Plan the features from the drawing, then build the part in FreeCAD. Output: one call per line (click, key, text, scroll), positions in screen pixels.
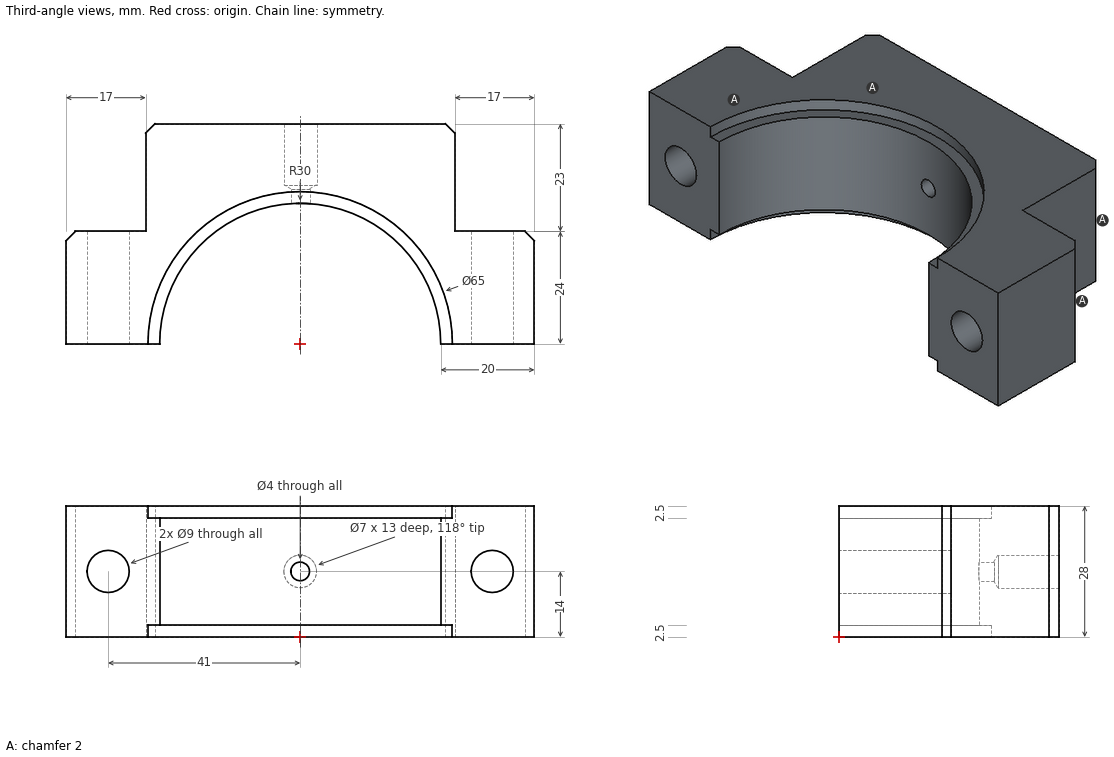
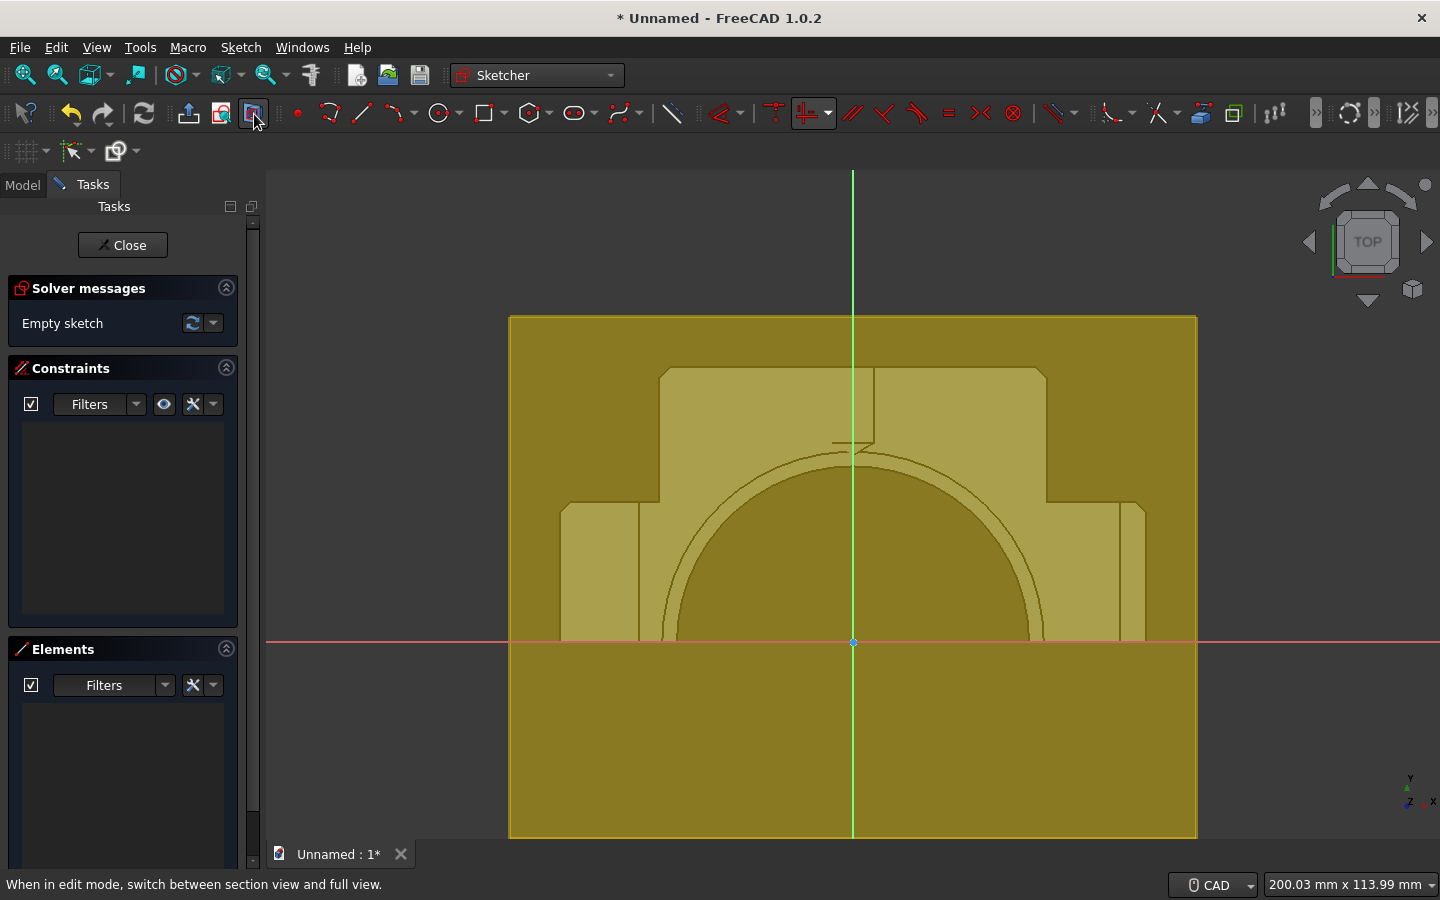
scroll(475, 198, down, 1)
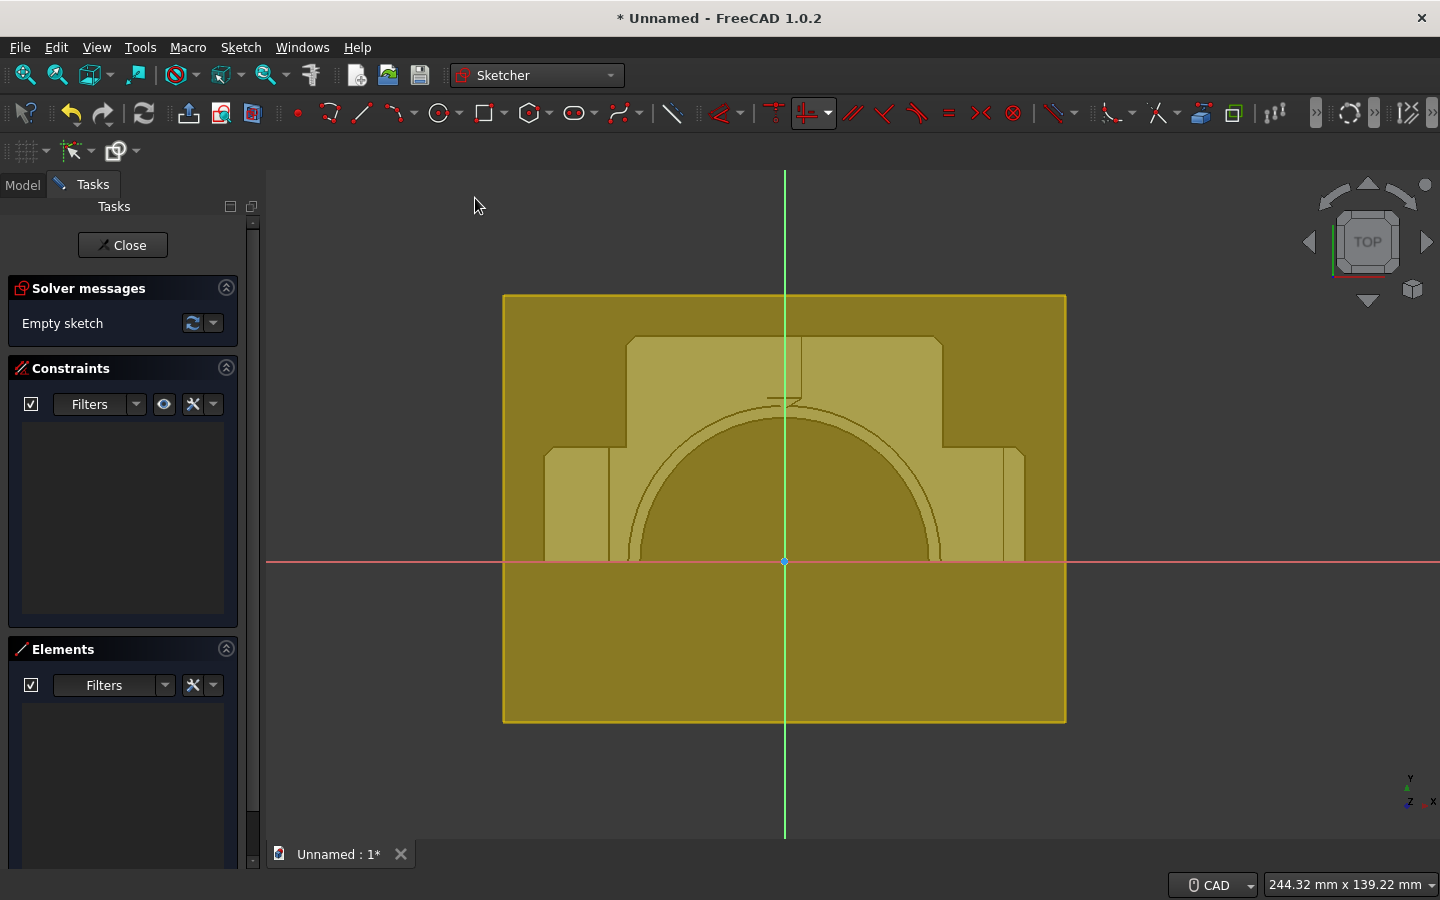
scroll(785, 679, up, 2)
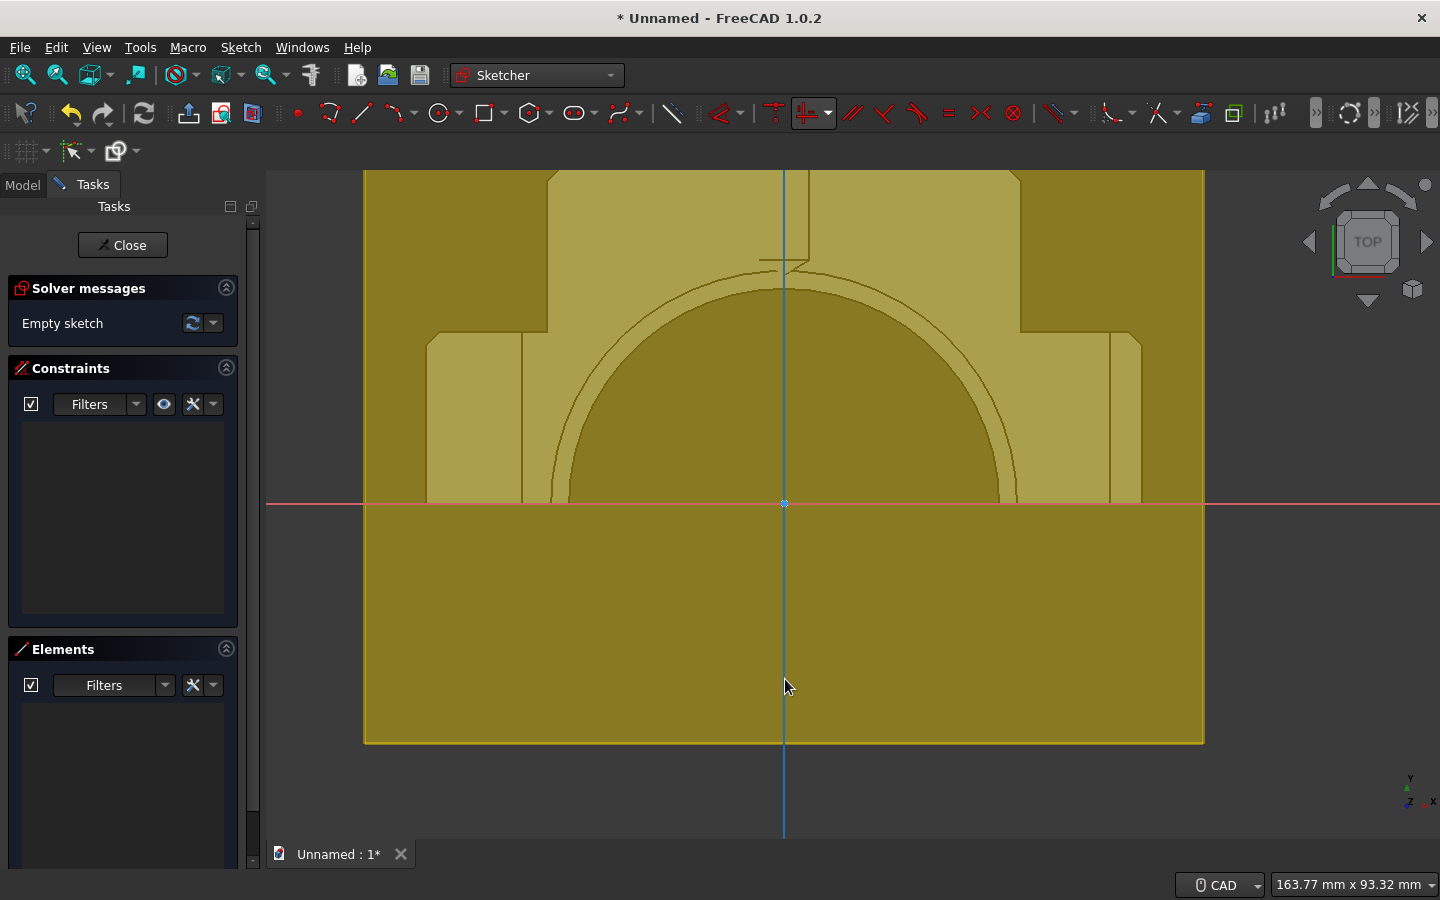
click(440, 114)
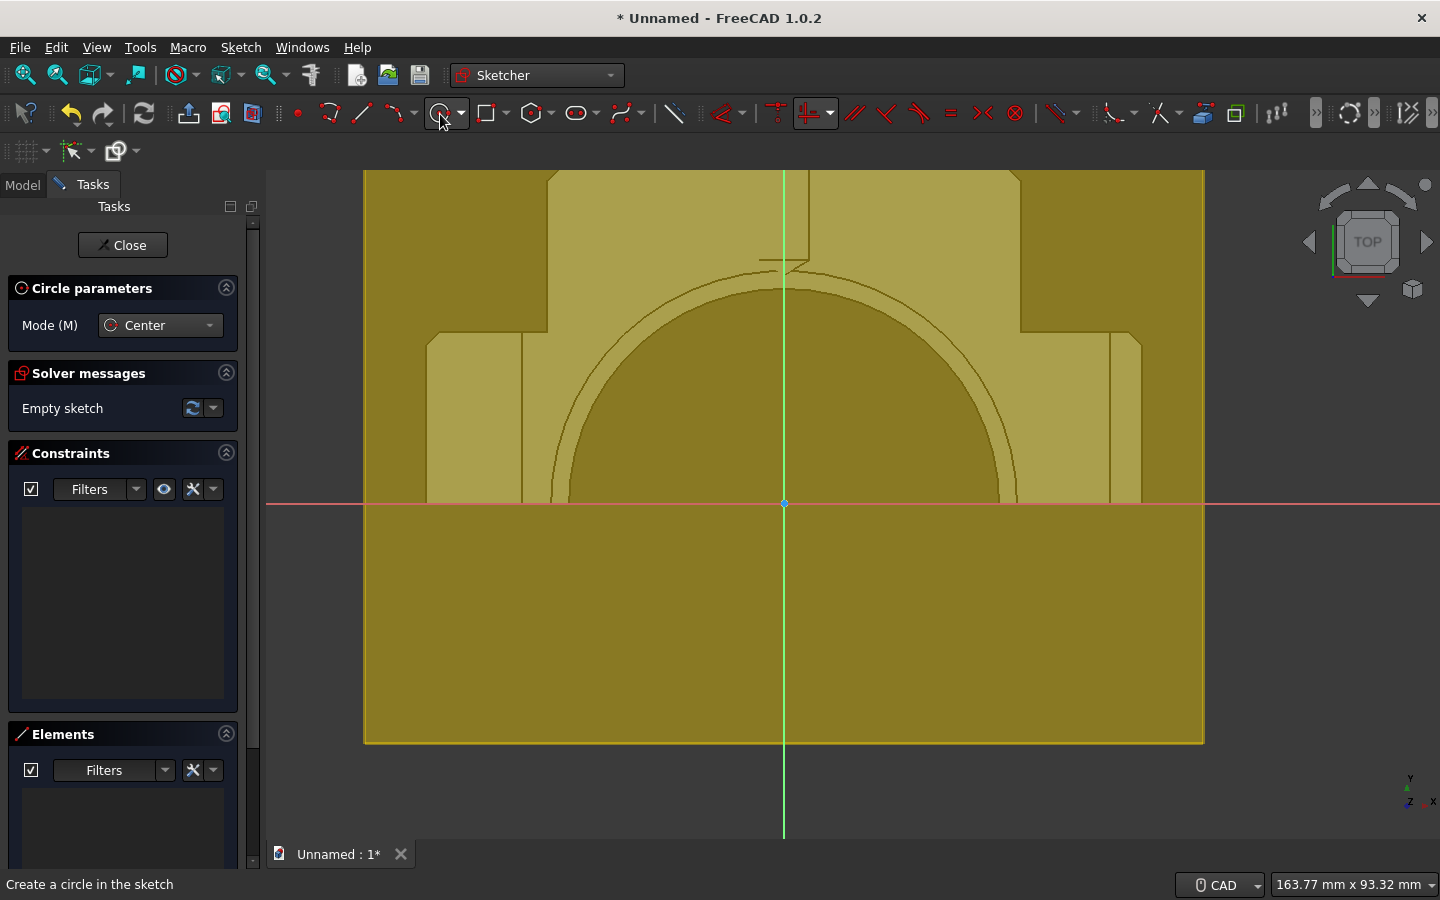
click(784, 504)
click(949, 339)
key(Escape)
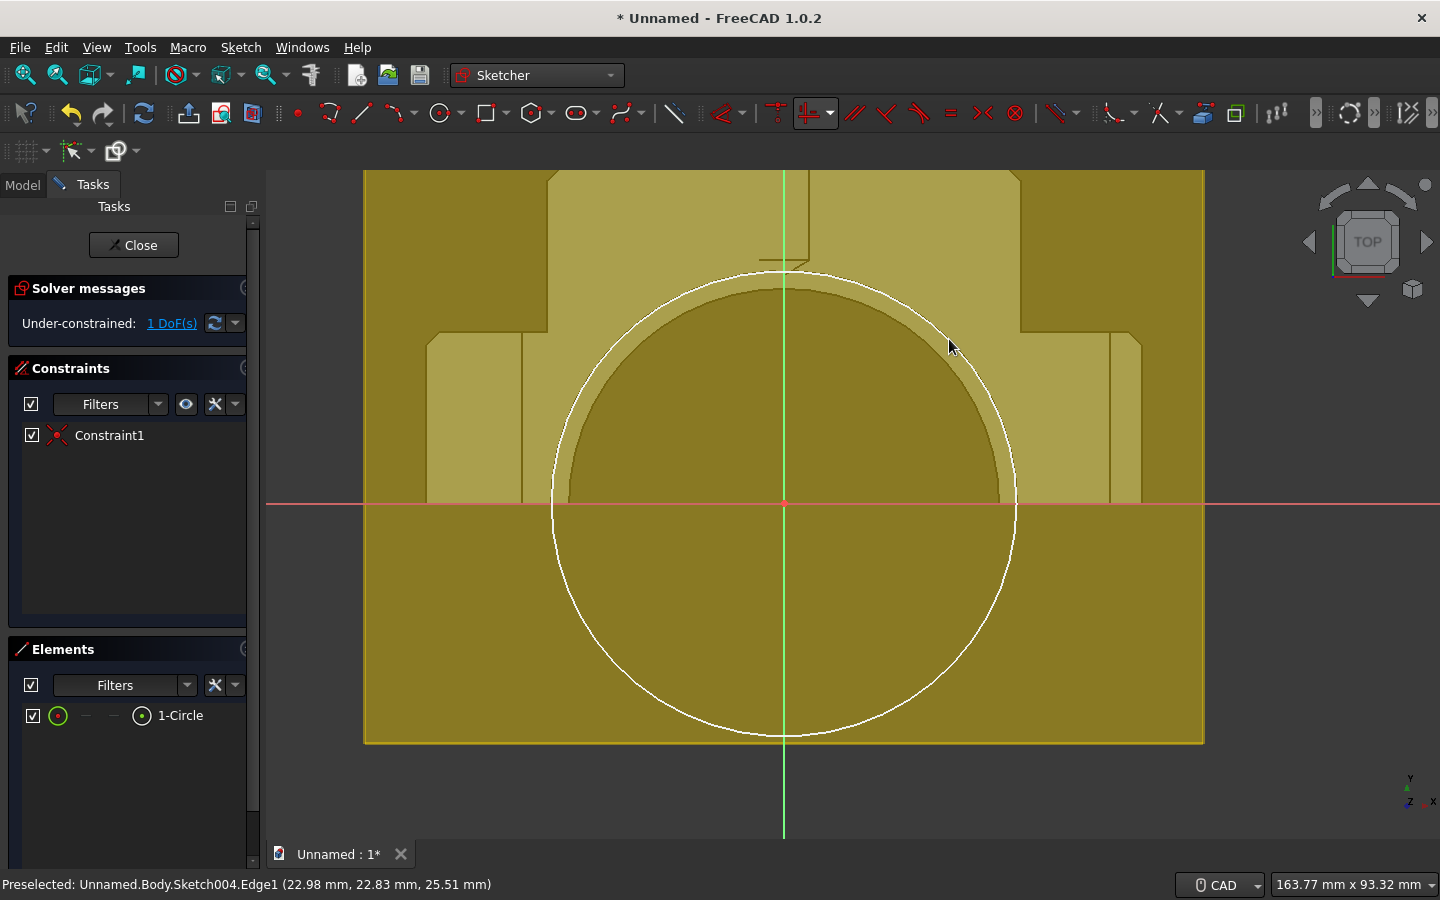
click(722, 114)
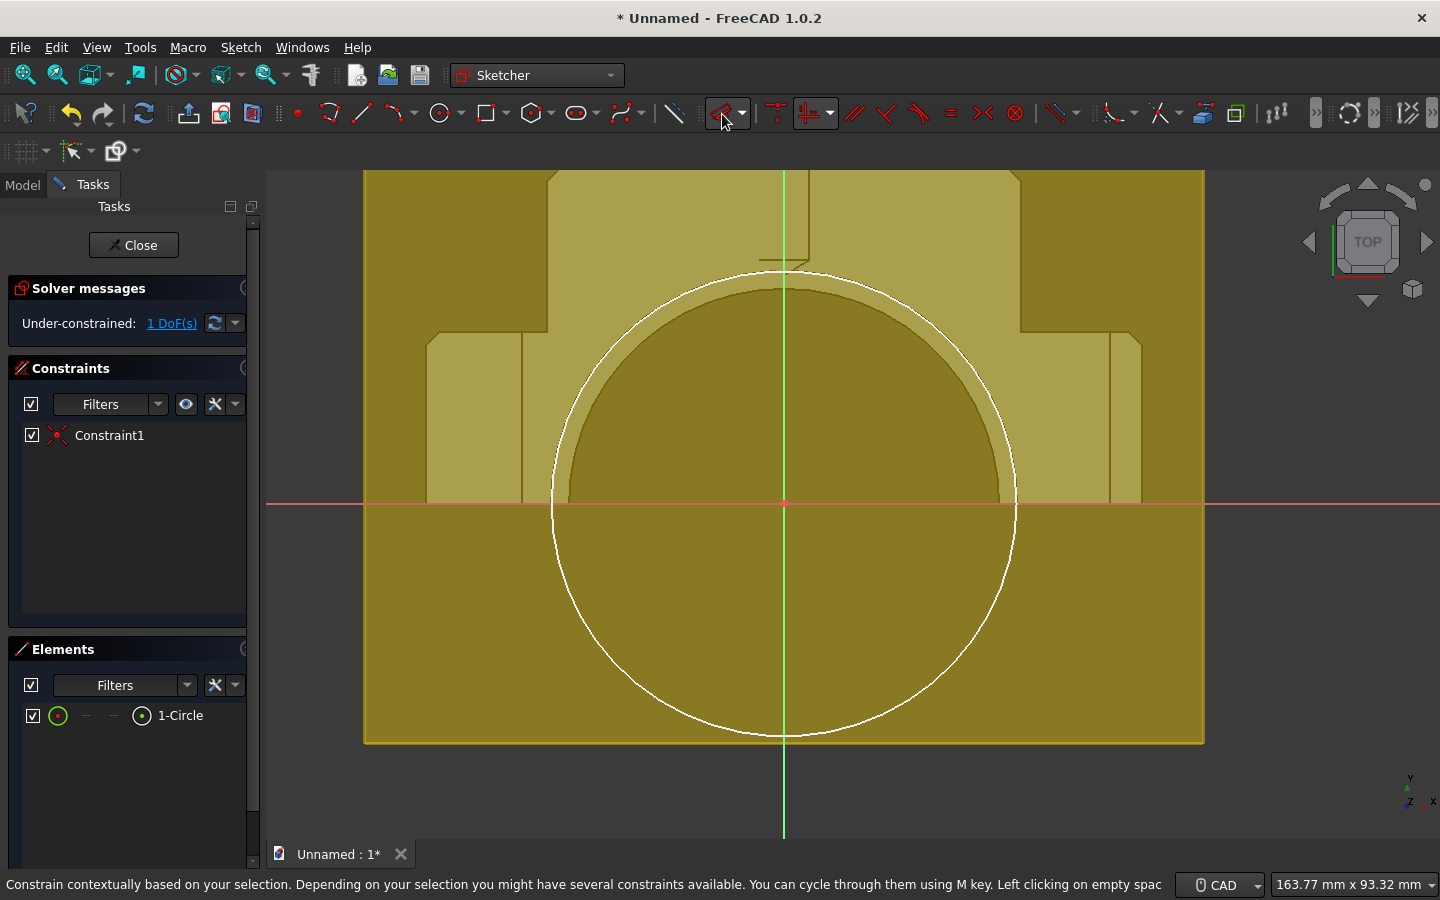
click(948, 339)
click(971, 316)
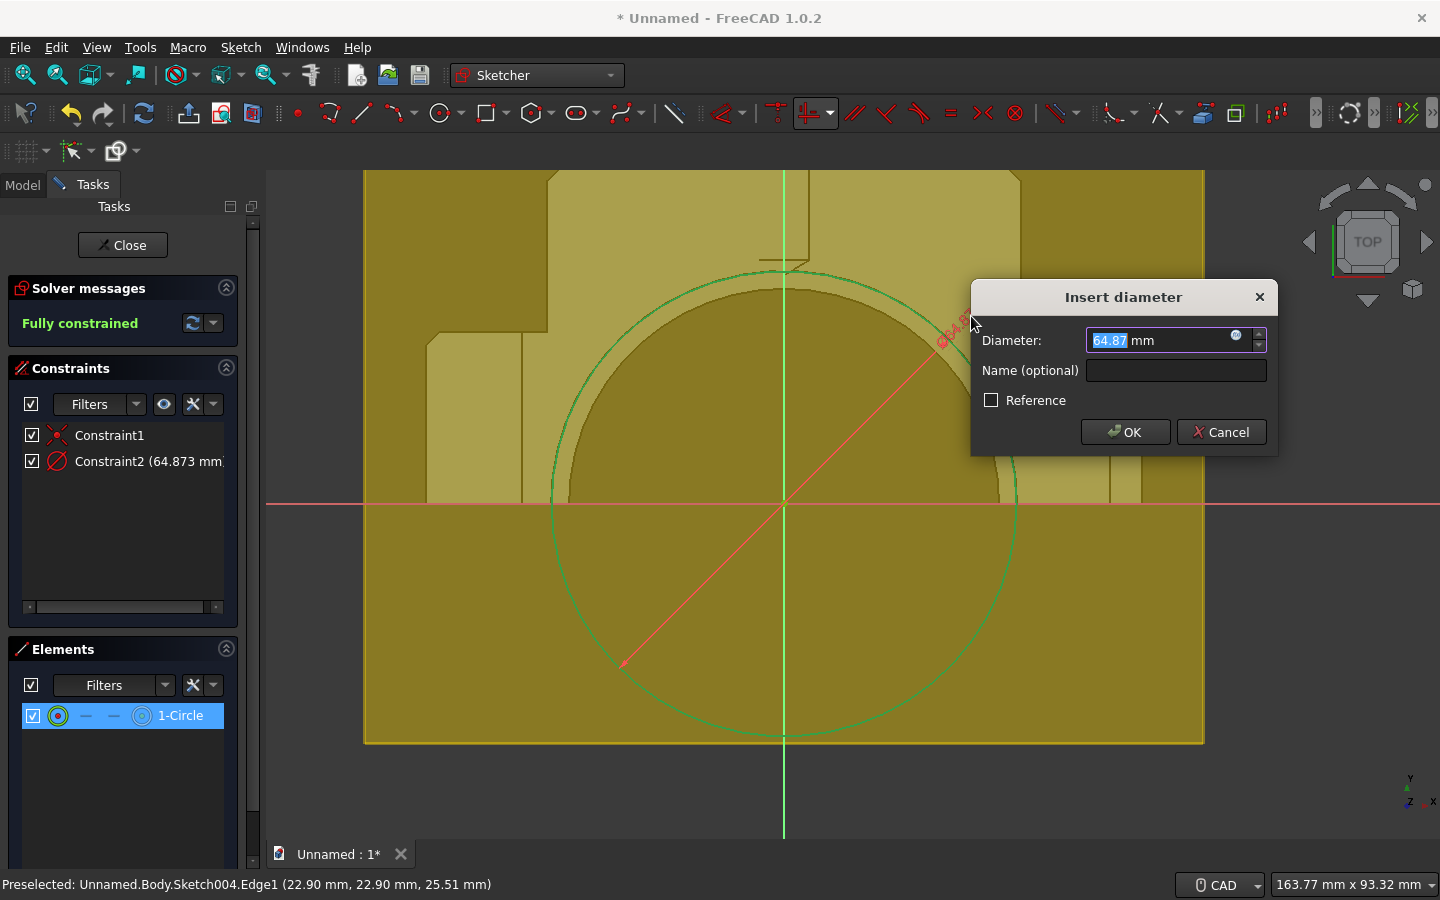
text(65)
key(Return)
key(Escape)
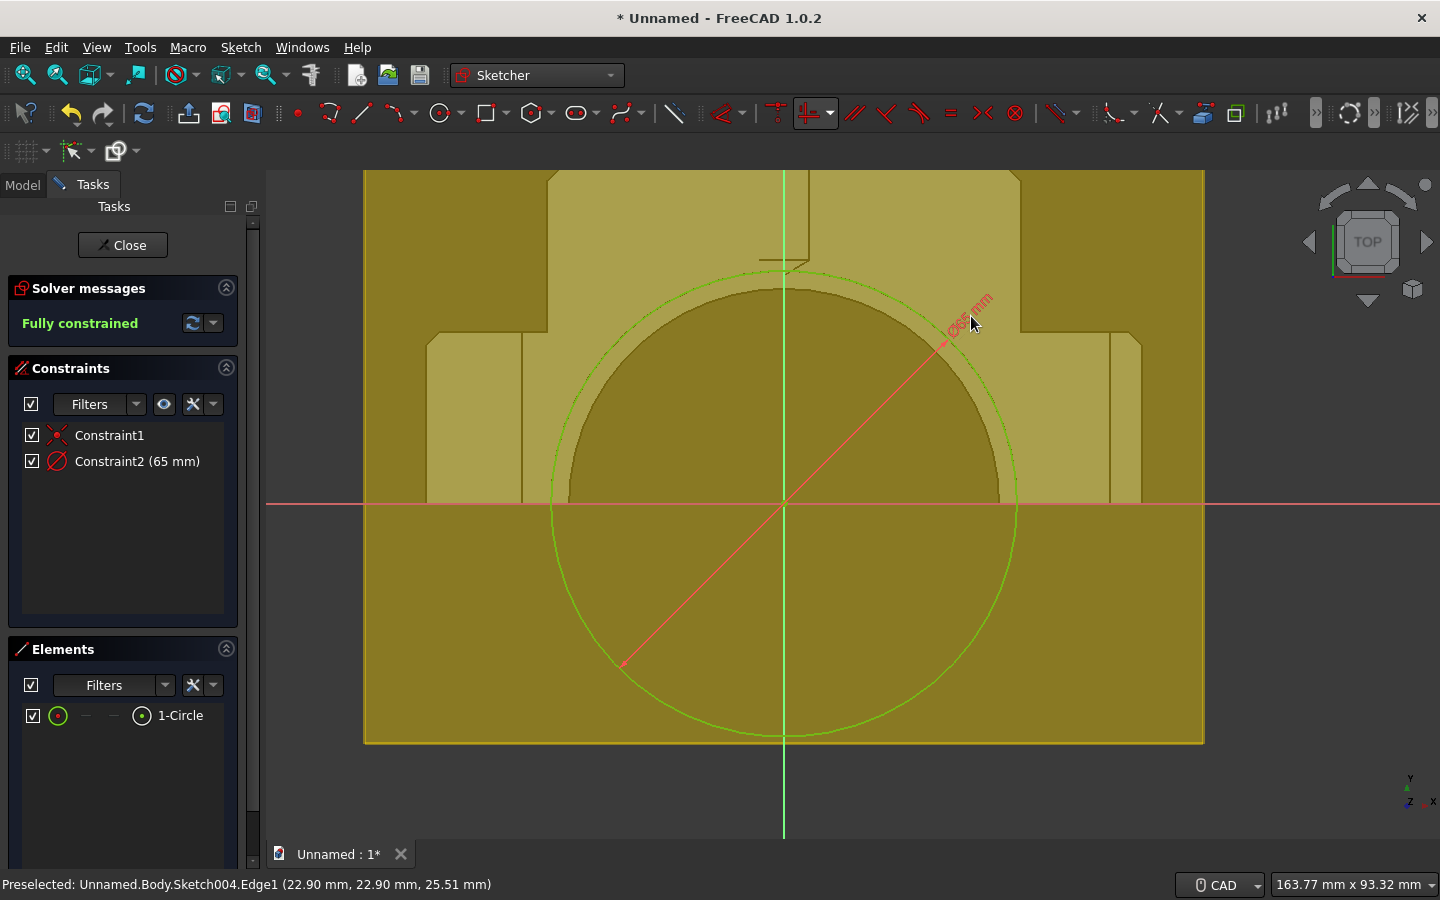
click(123, 245)